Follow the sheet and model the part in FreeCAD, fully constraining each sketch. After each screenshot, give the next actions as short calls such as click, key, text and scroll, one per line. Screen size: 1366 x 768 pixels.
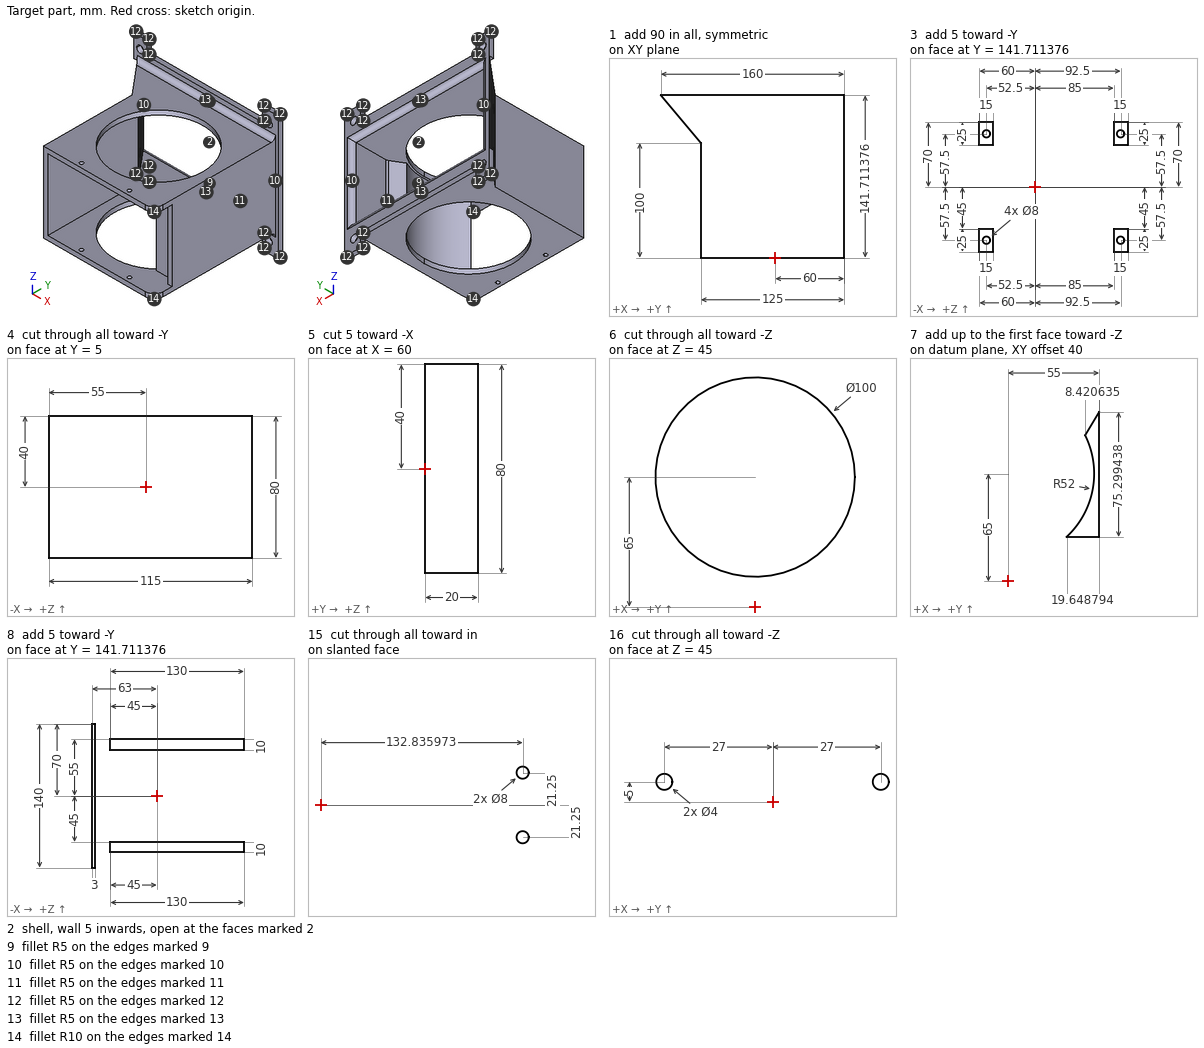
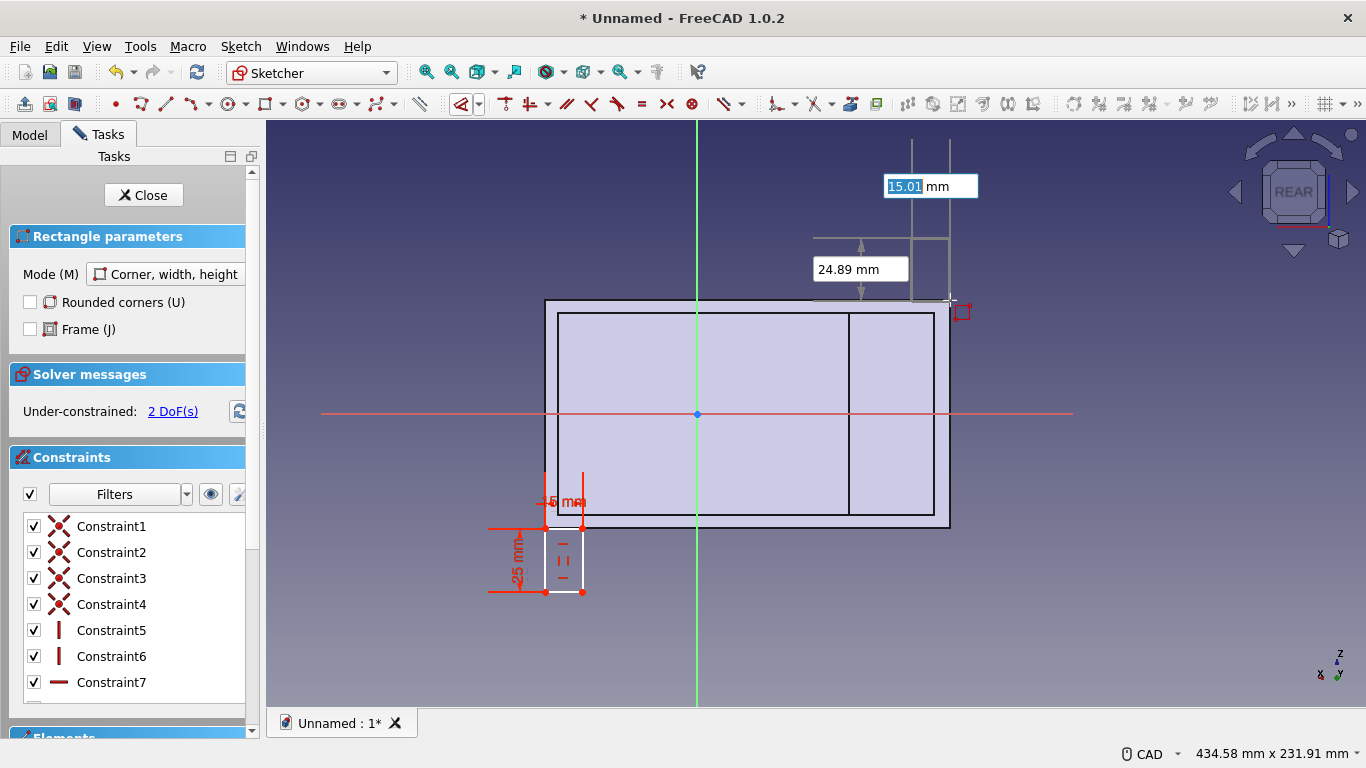
text(15)
key(Tab)
text(25)
key(Return)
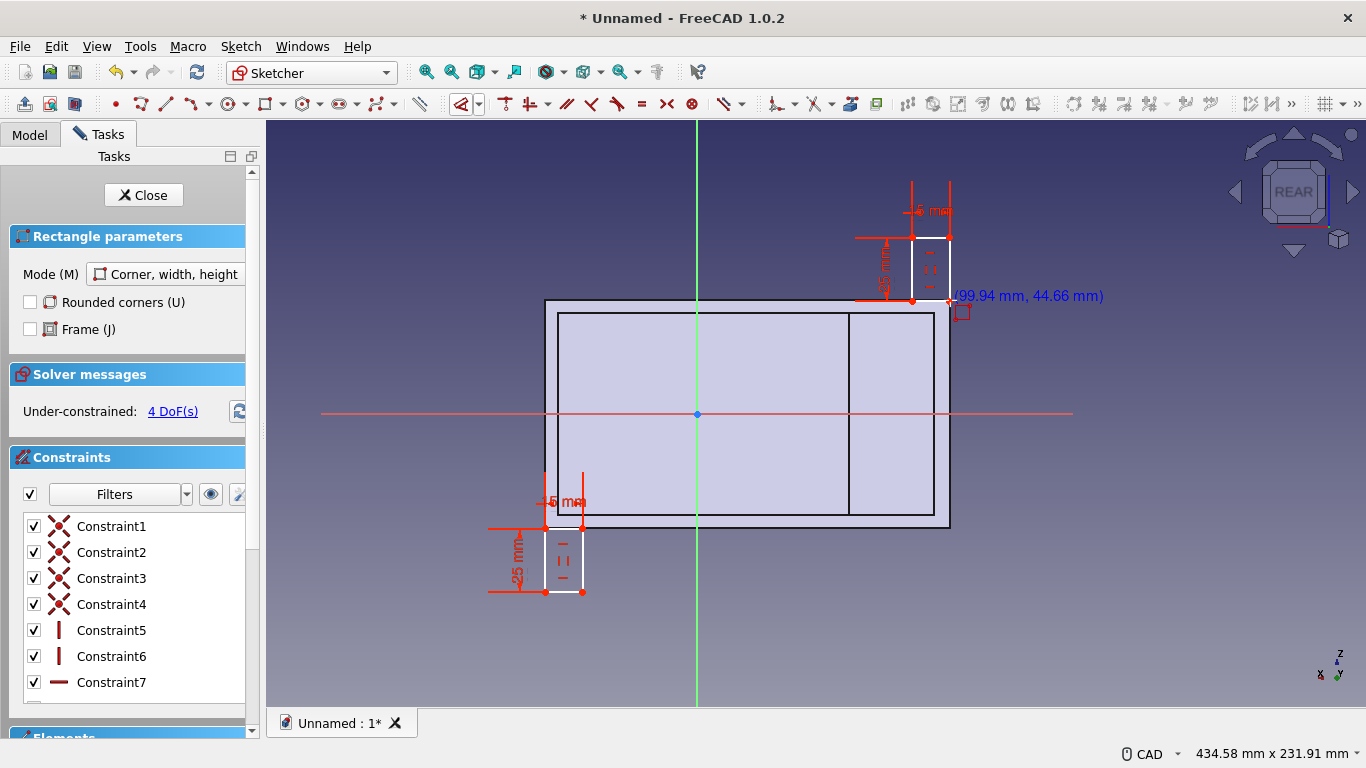
click(545, 237)
move(583, 300)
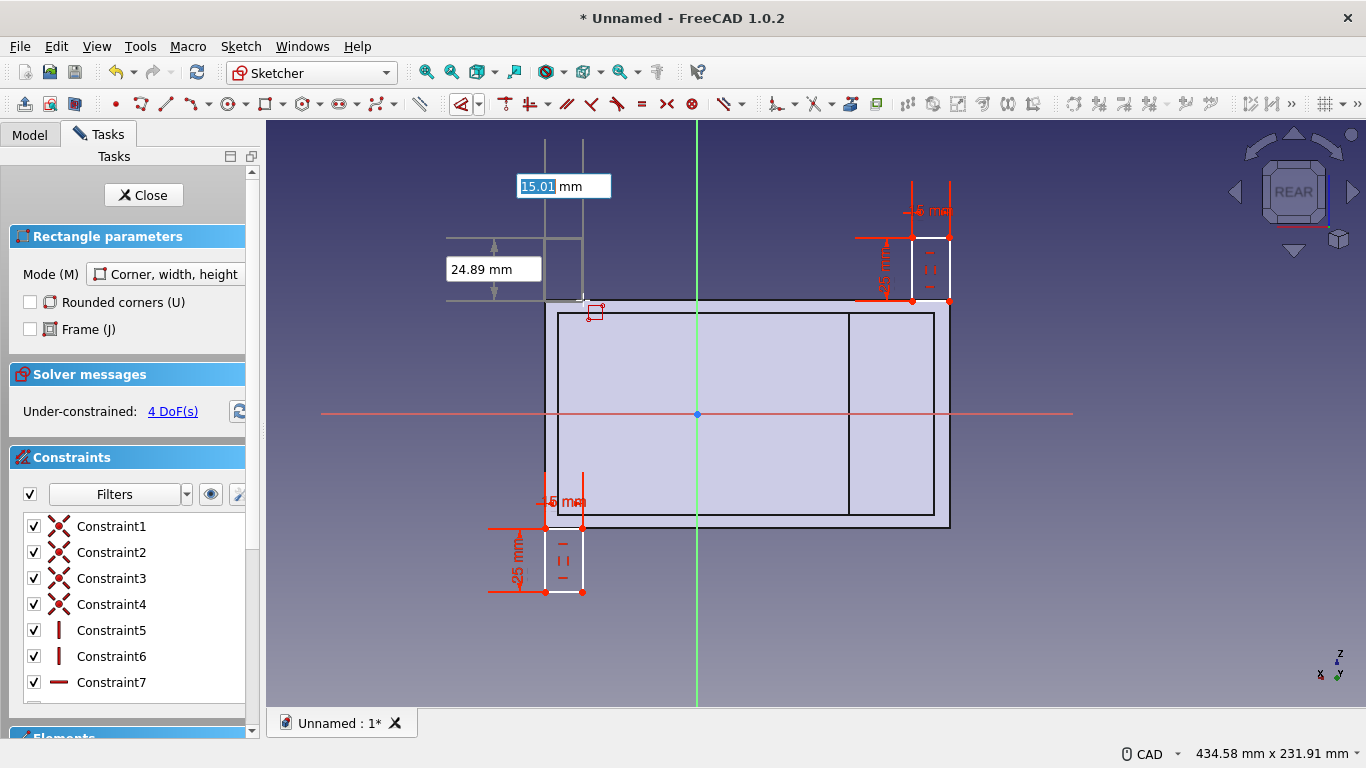
text(15)
key(Tab)
text(25)
key(Return)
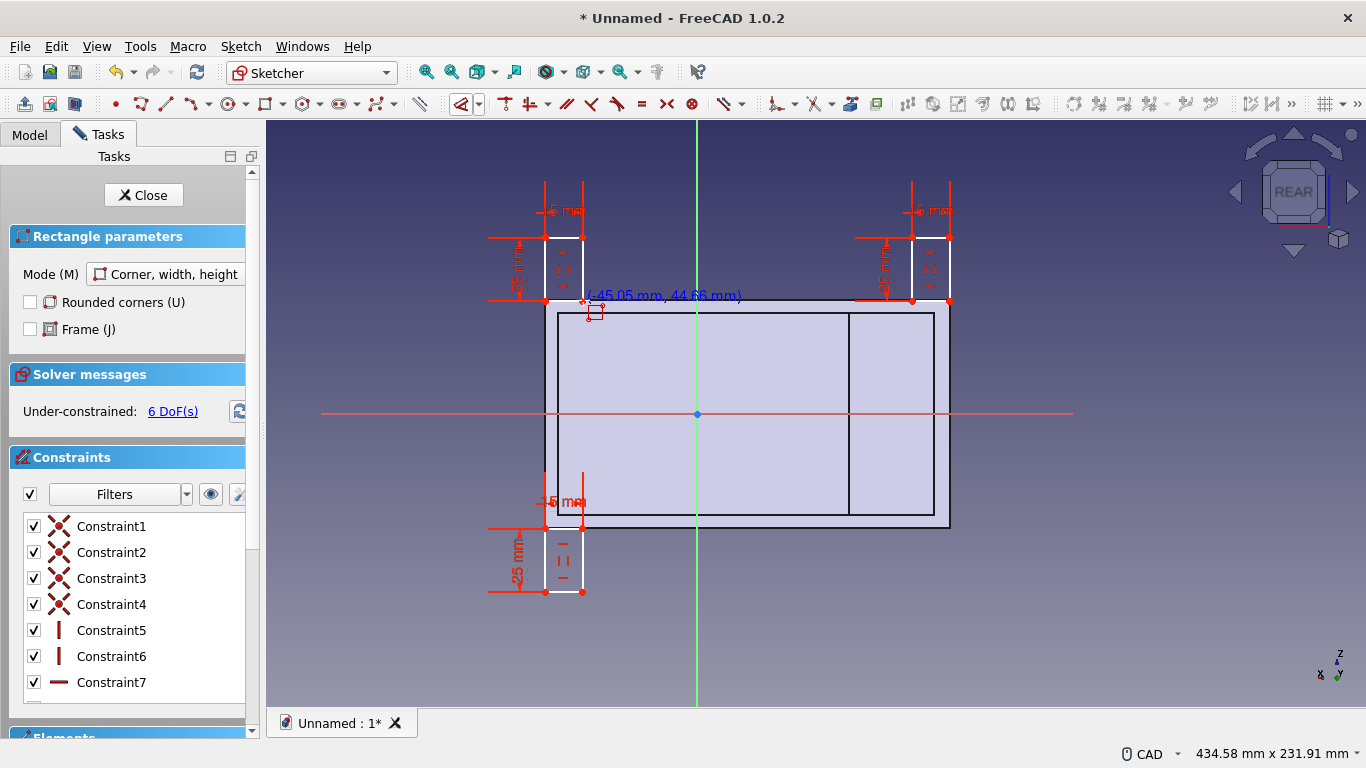
click(912, 528)
move(950, 591)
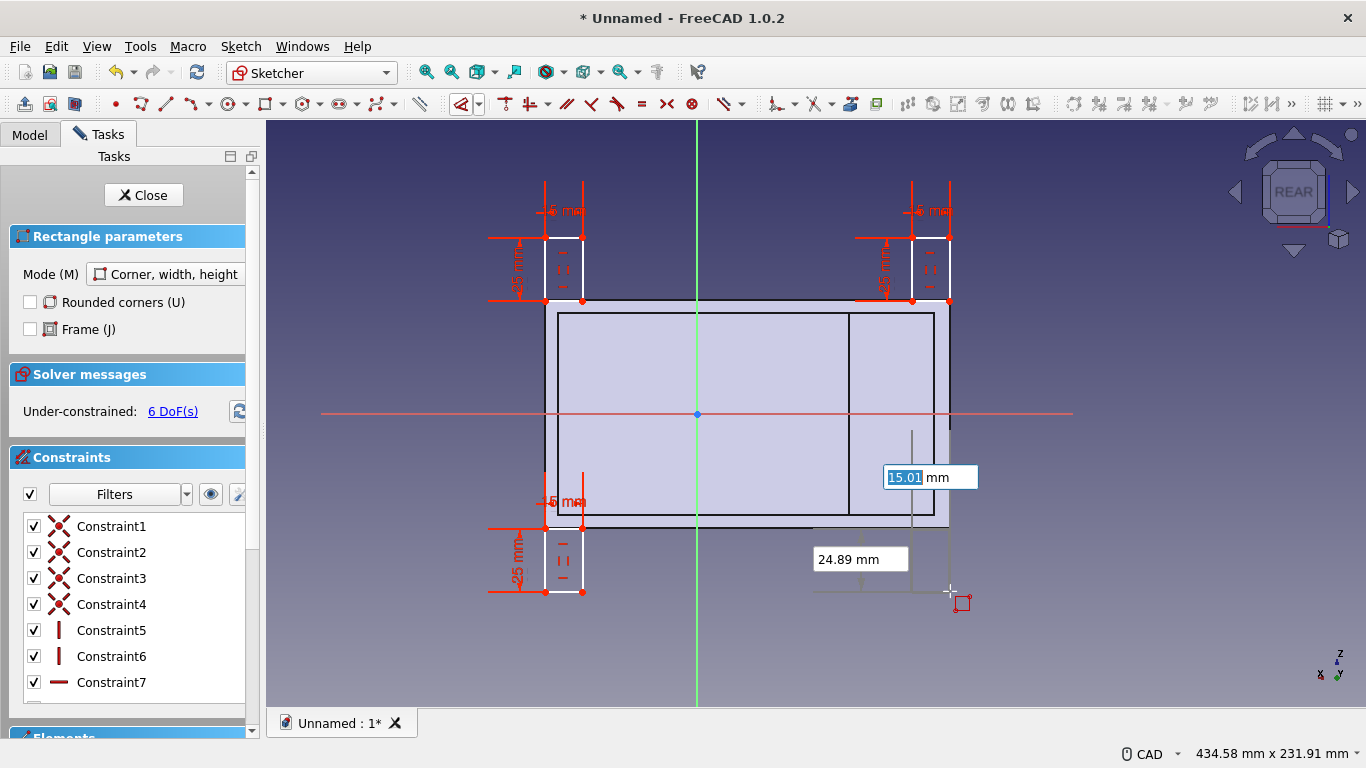
text(15)
key(Tab)
text(25)
key(Return)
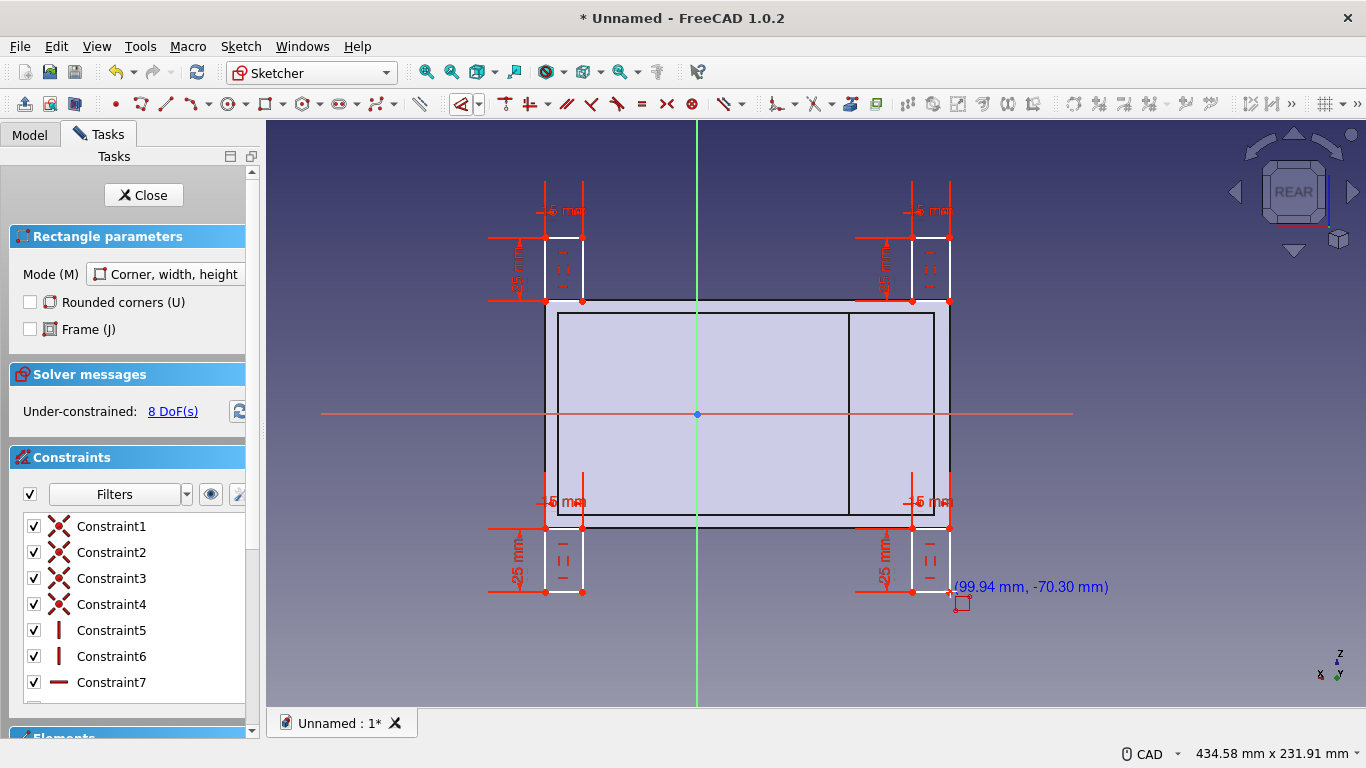
key(g)
key(c)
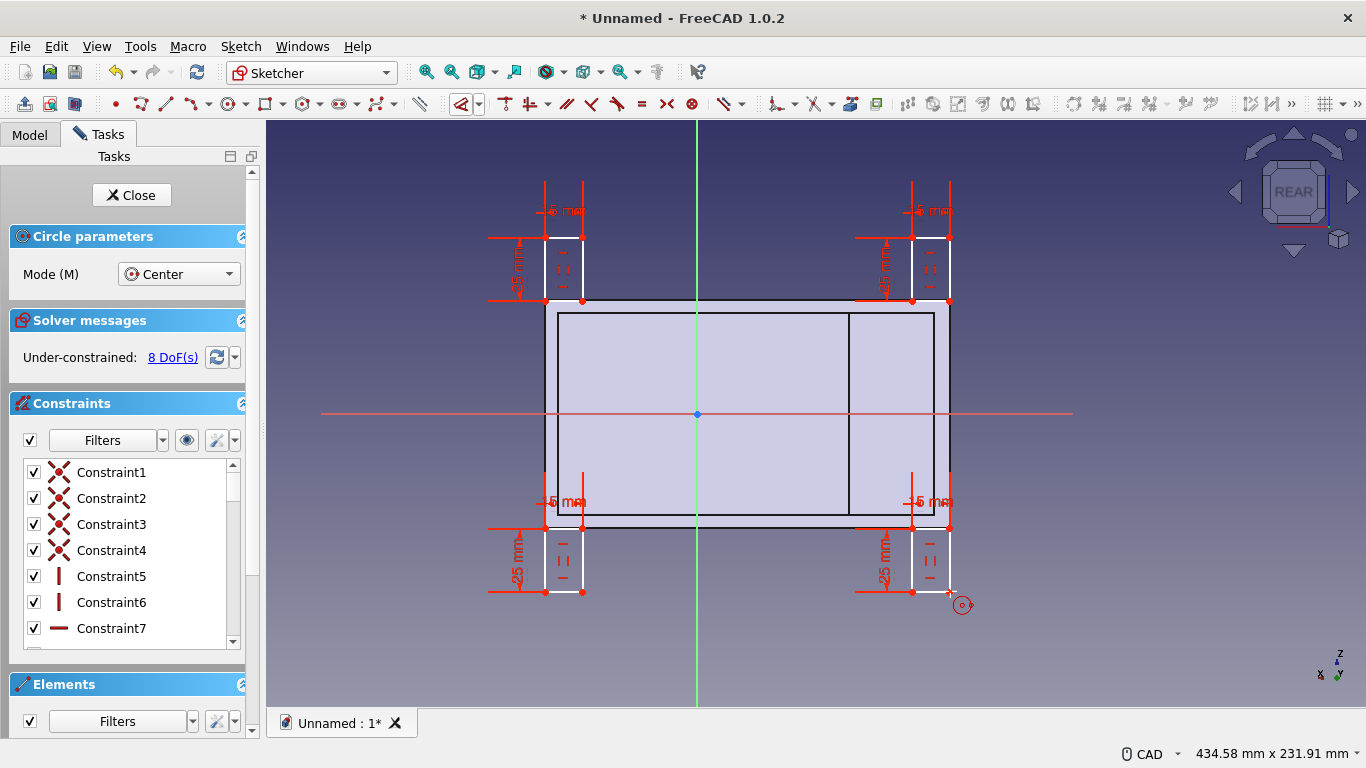
scroll(564, 560, up, 5)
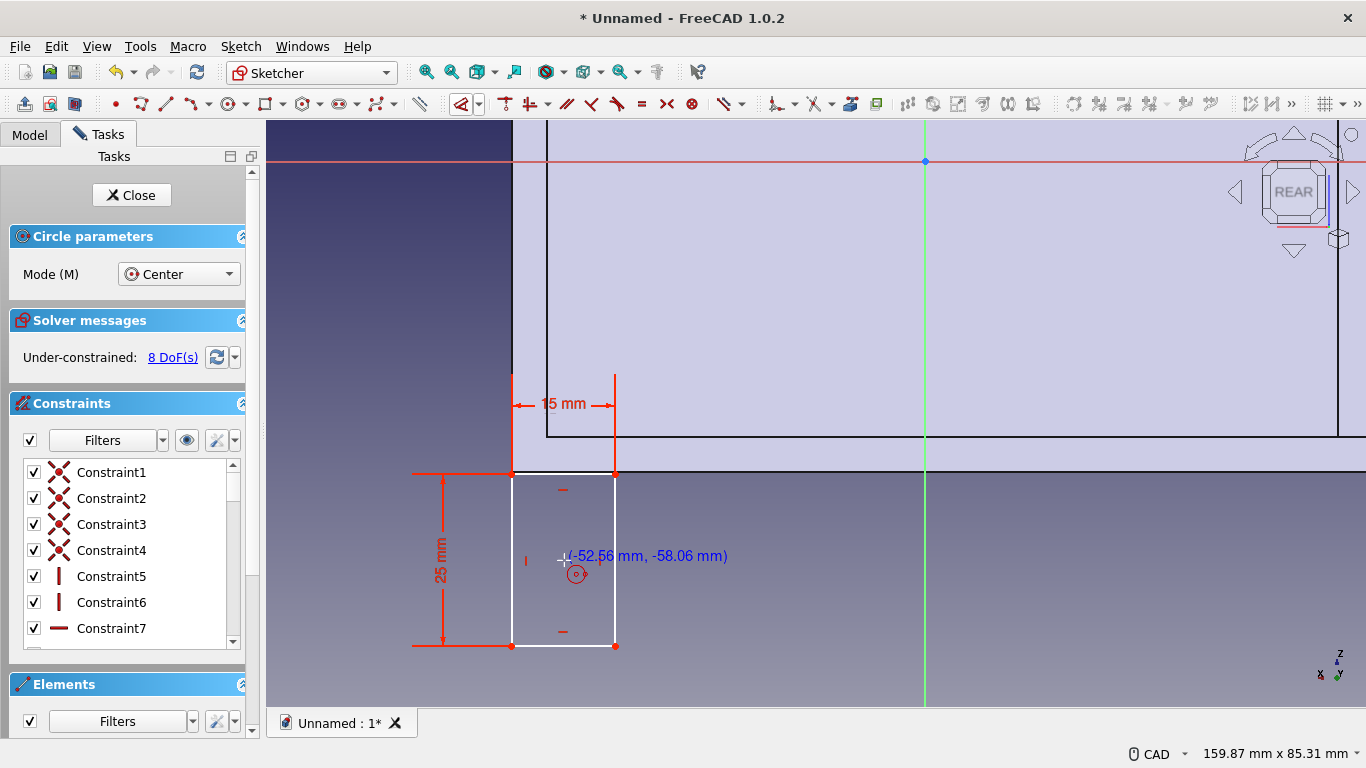
click(564, 558)
move(583, 538)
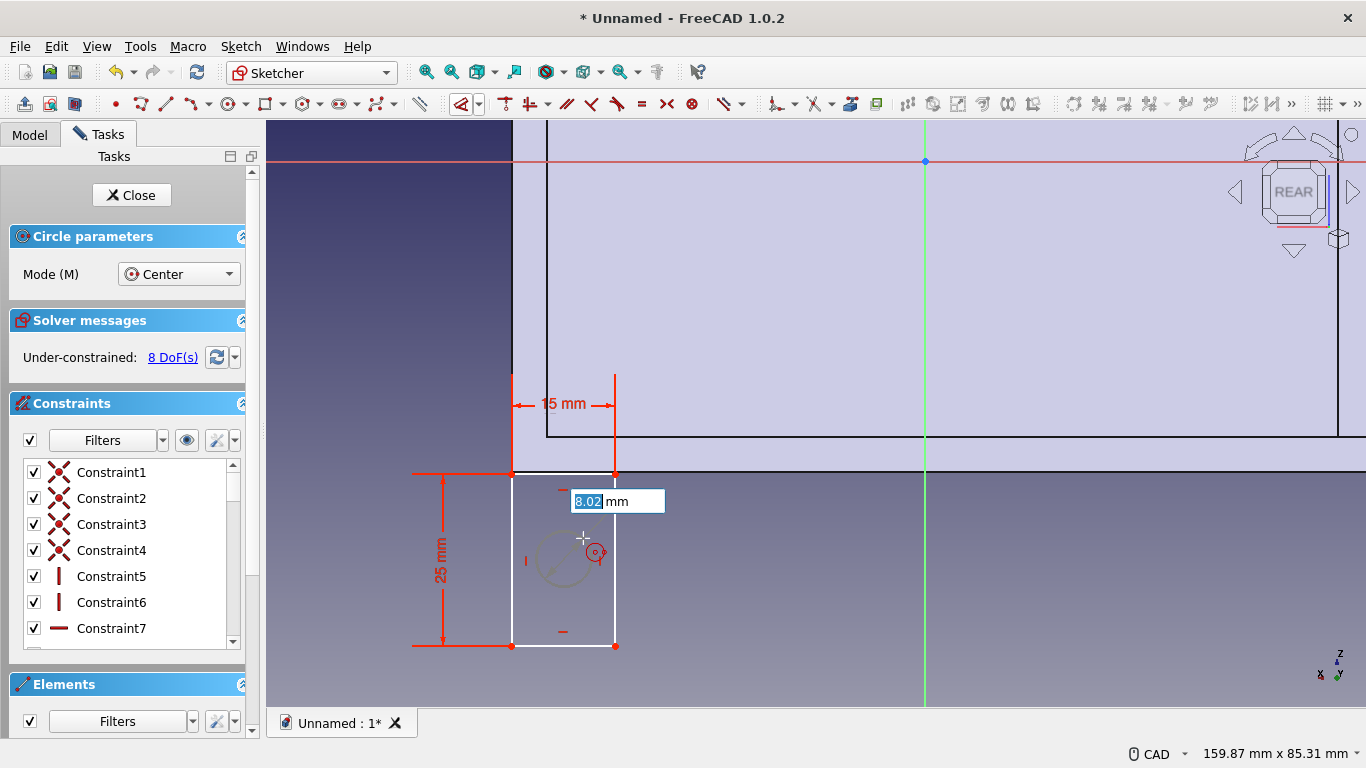
text(8)
key(Return)